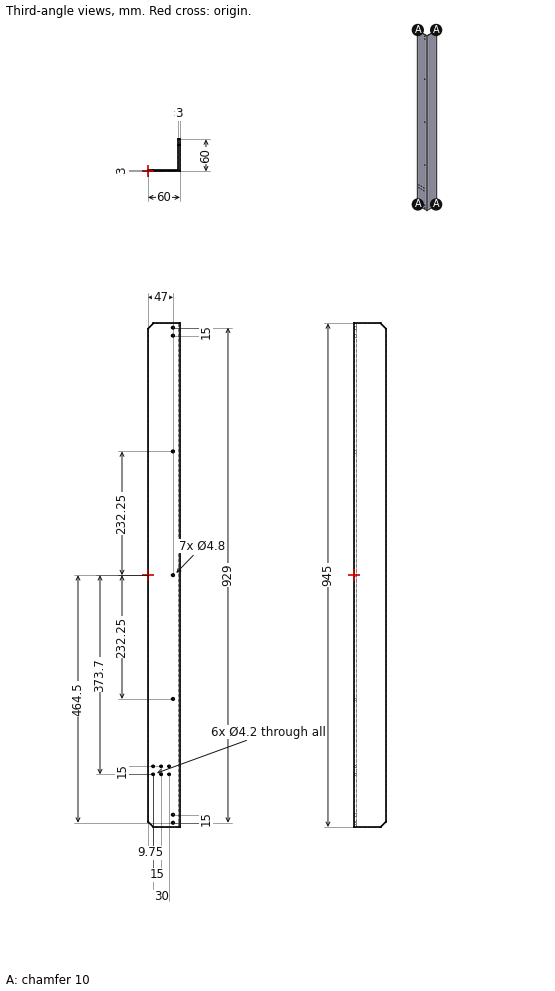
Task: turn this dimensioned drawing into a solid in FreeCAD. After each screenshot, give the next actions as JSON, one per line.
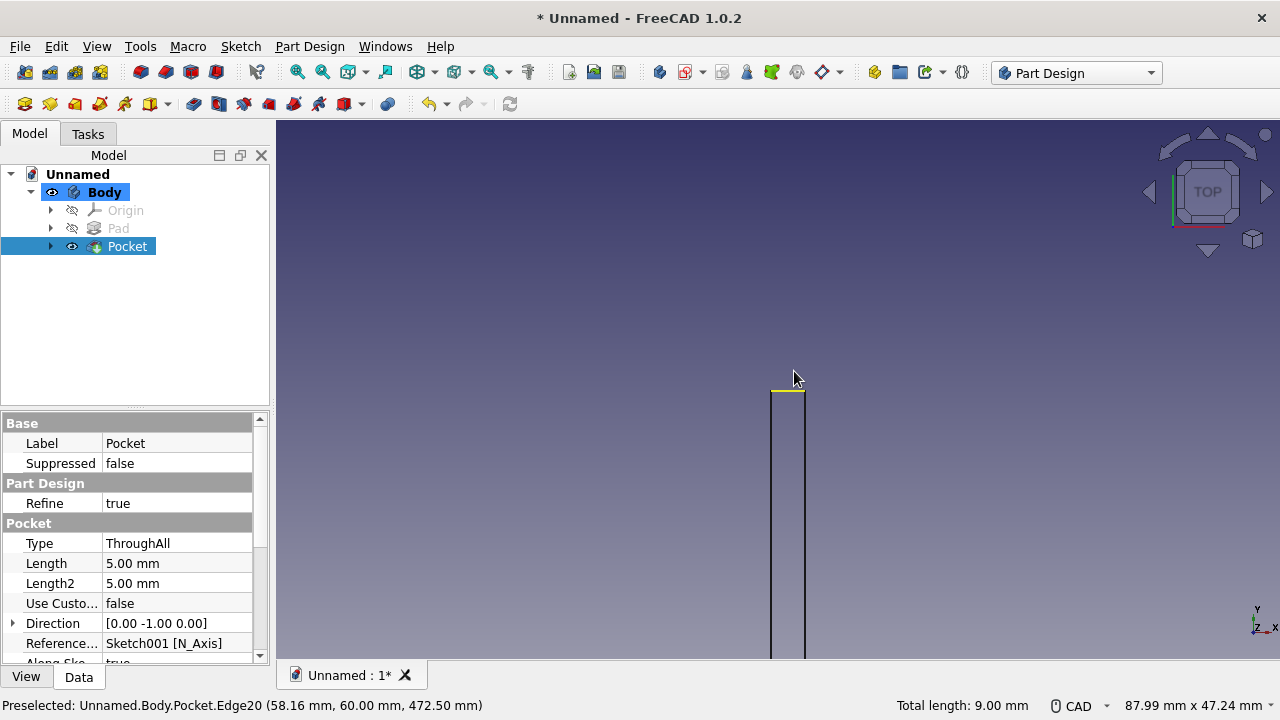
{"action": "left_click", "coordinate": [298, 72]}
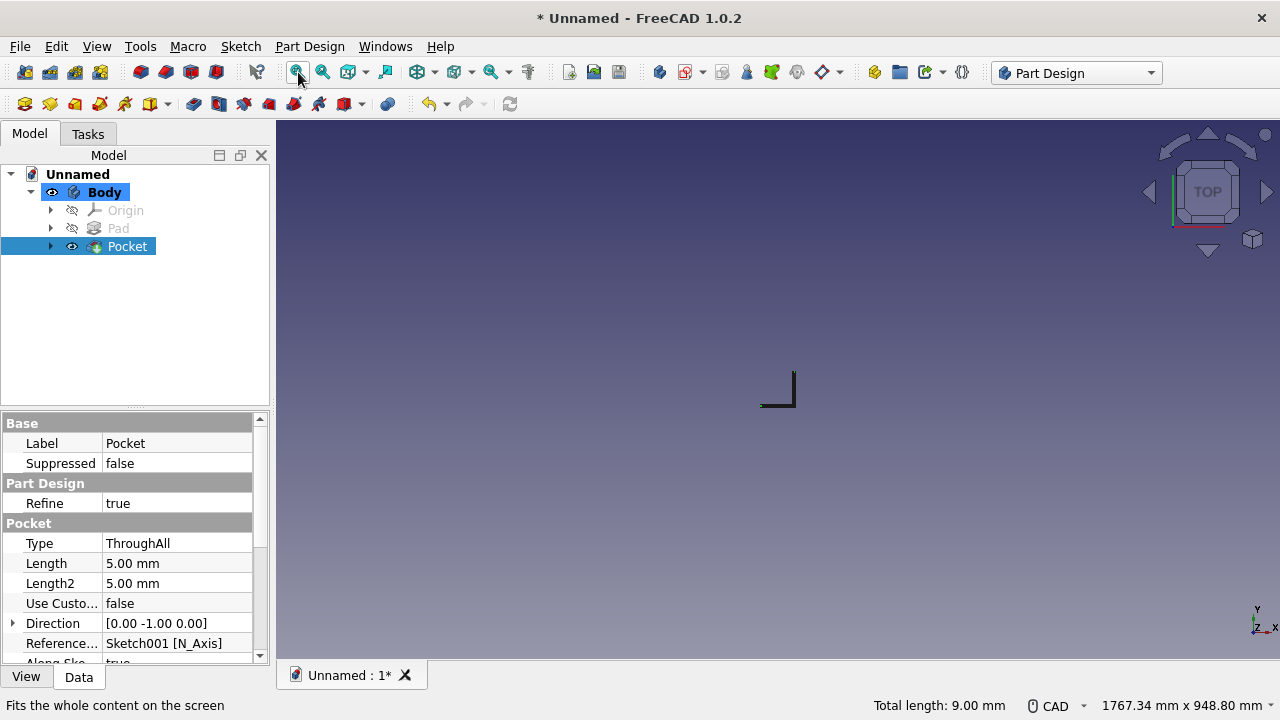
{"action": "key", "text": "1"}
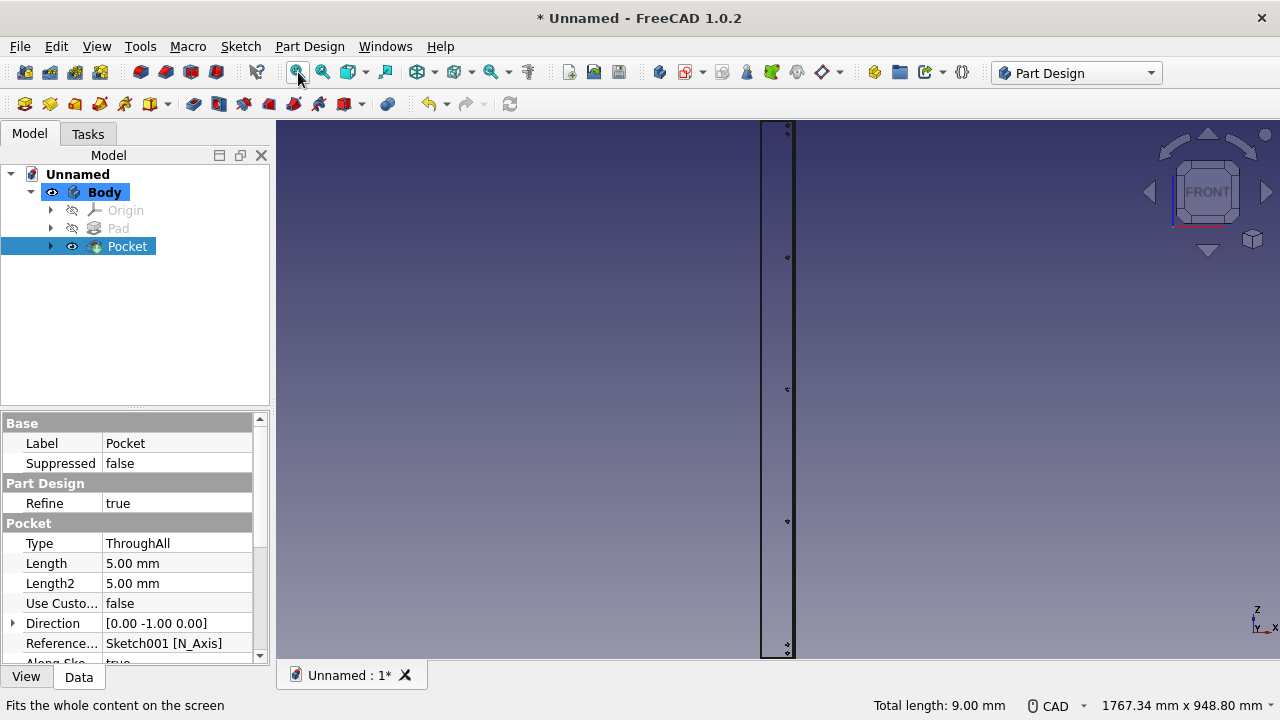
{"action": "key", "text": "3"}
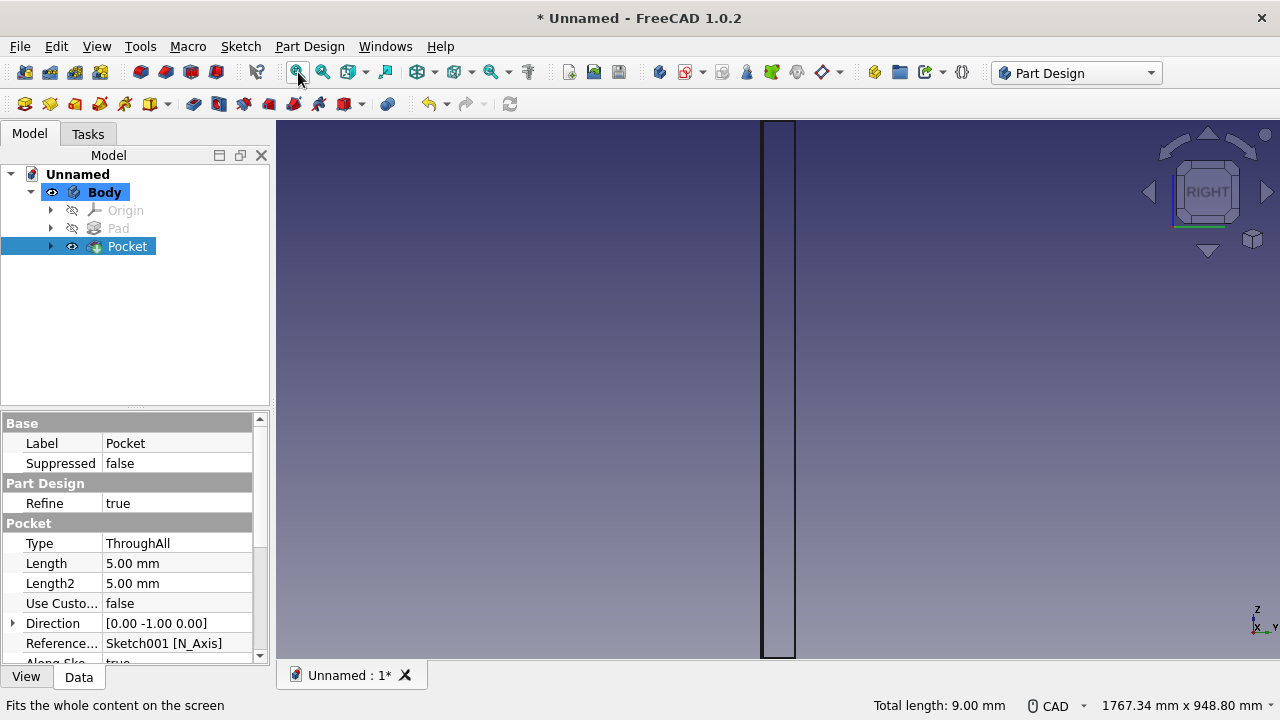
{"action": "key", "text": "5"}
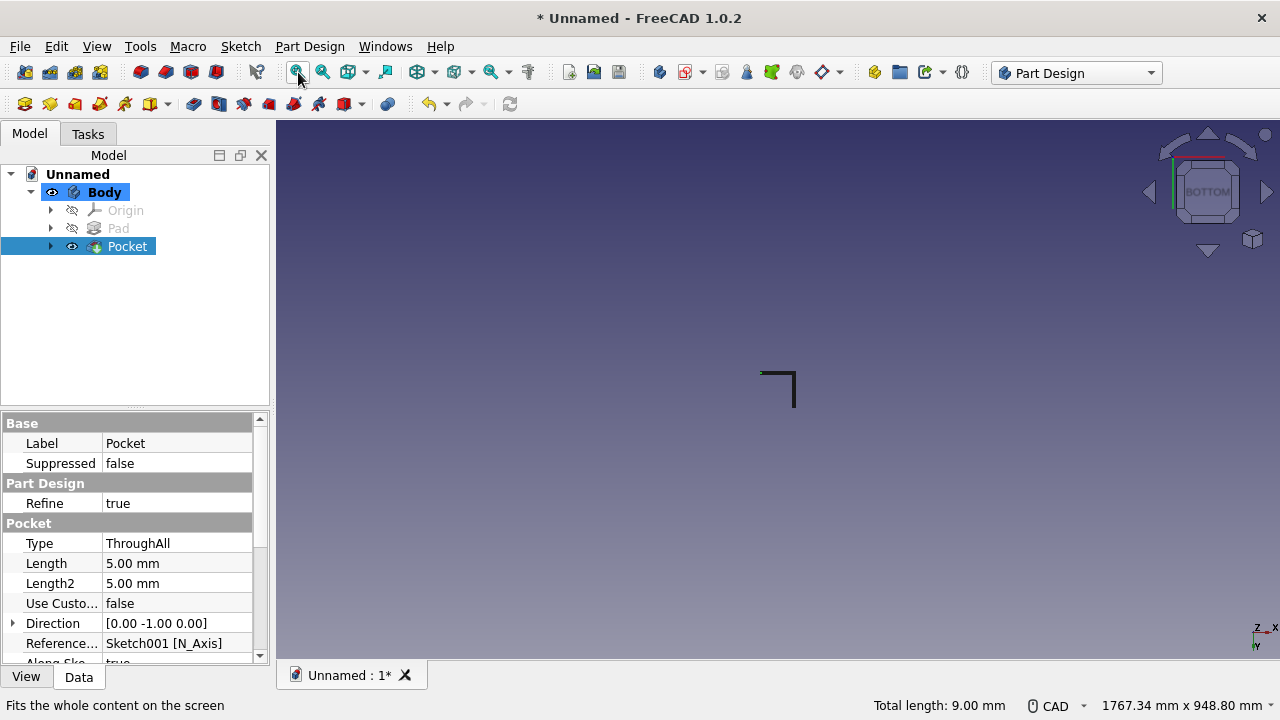
{"action": "left_click", "coordinate": [298, 72]}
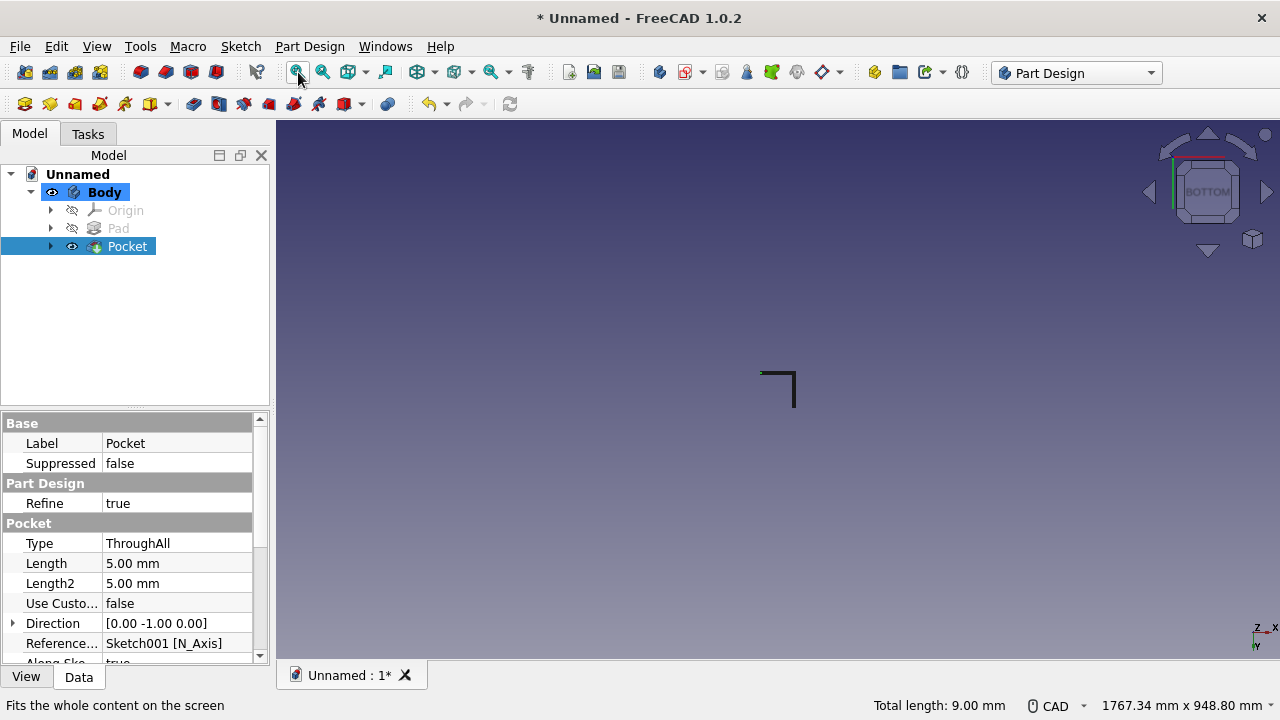
{"action": "scroll", "coordinate": [794, 406], "scroll_direction": "up", "scroll_amount": 15}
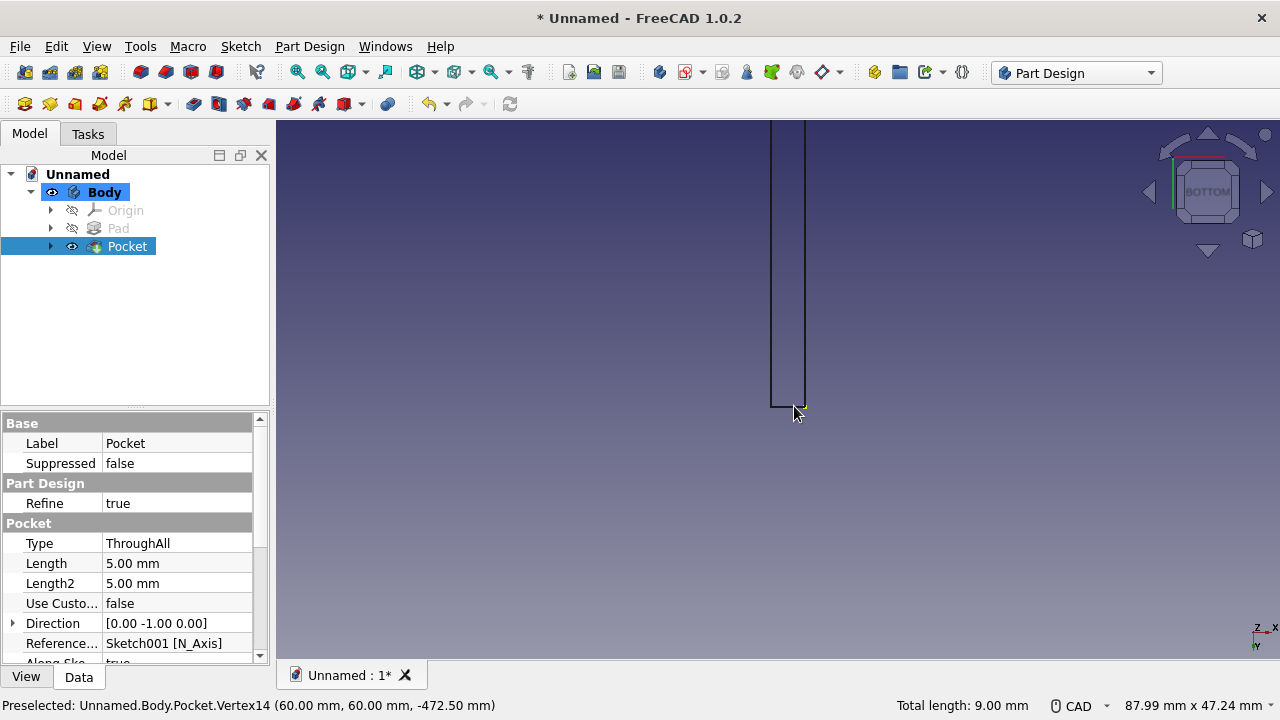
{"action": "left_click", "coordinate": [788, 406], "text": "ctrl"}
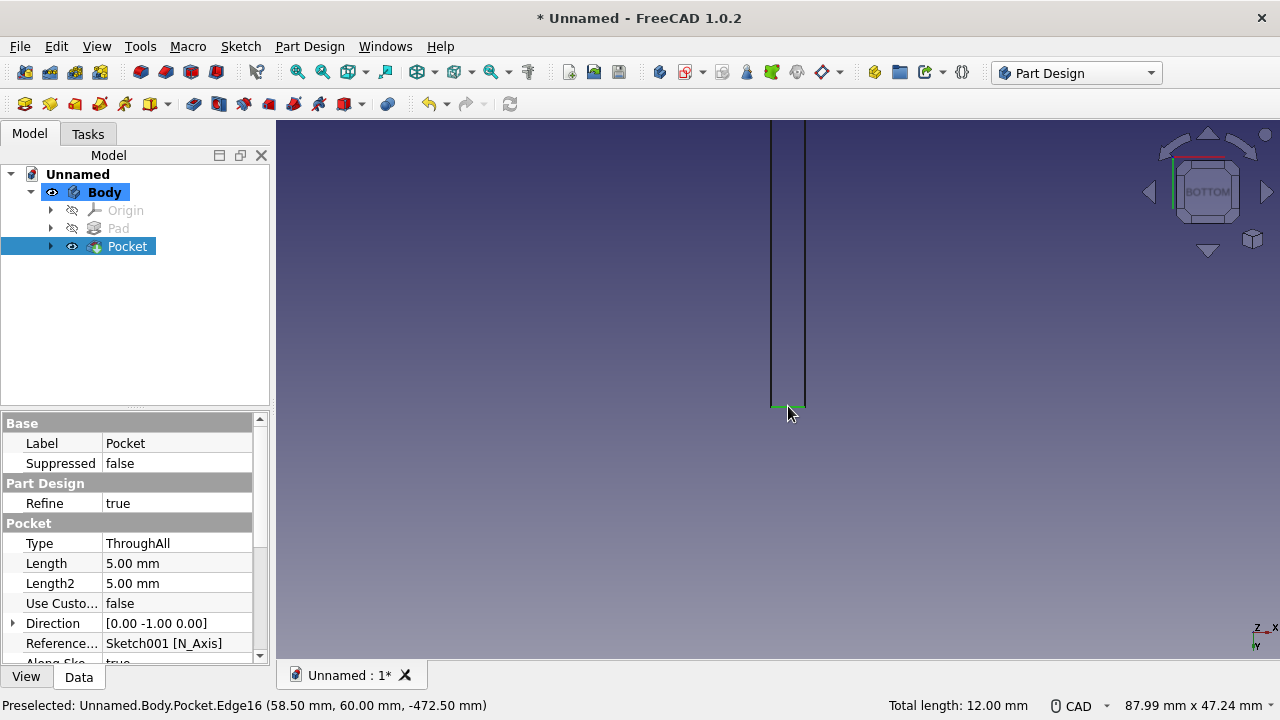
{"action": "key", "text": "v 1"}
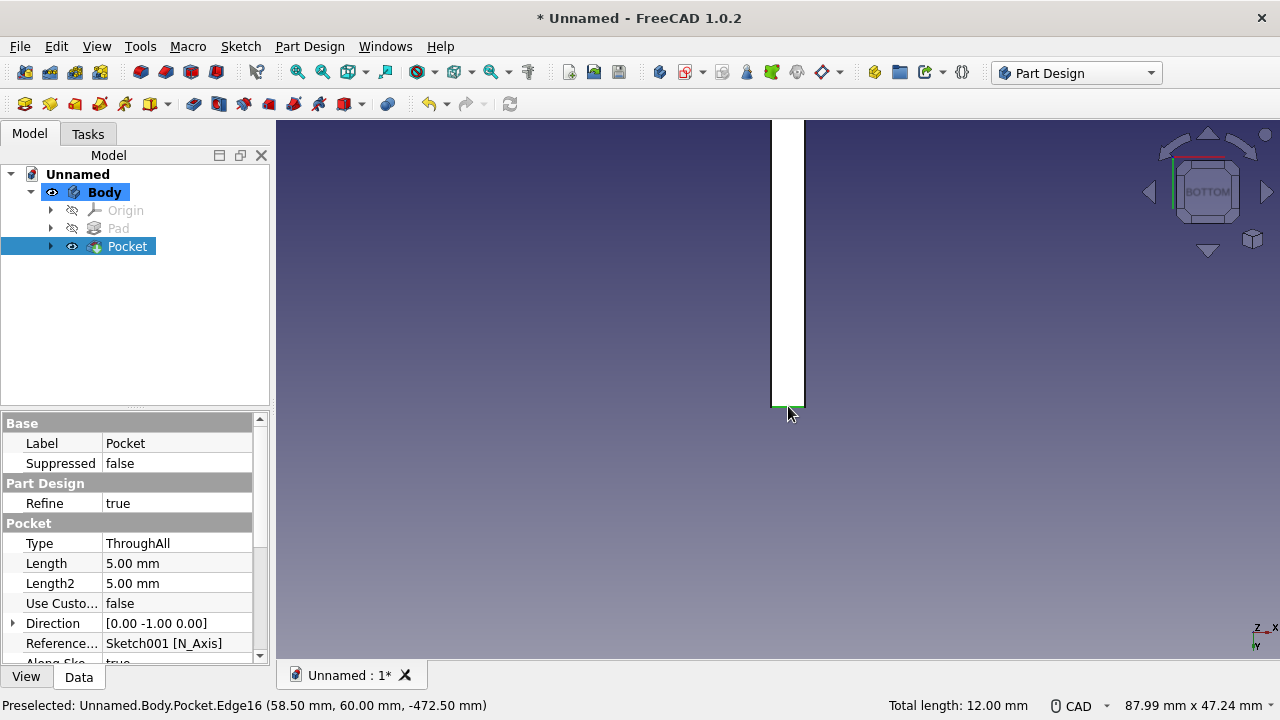
{"action": "left_click", "coordinate": [166, 72]}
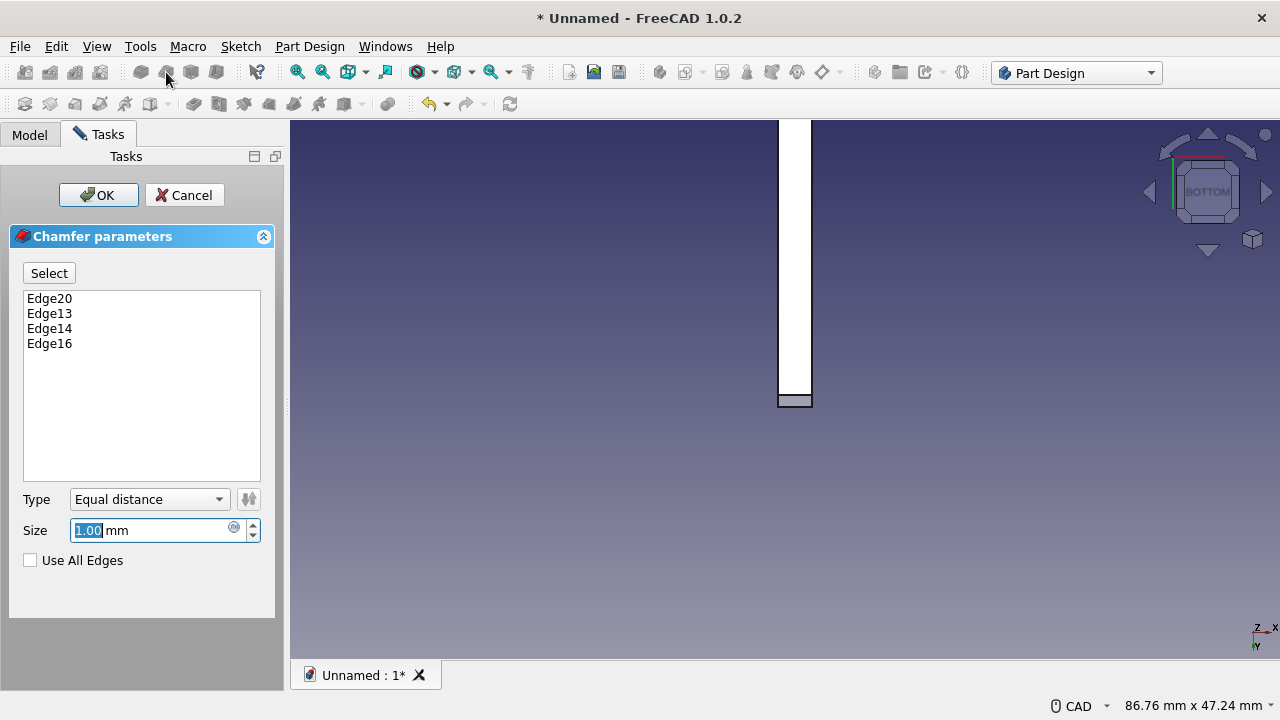
{"action": "type", "text": "10"}
{"action": "key", "text": "Tab"}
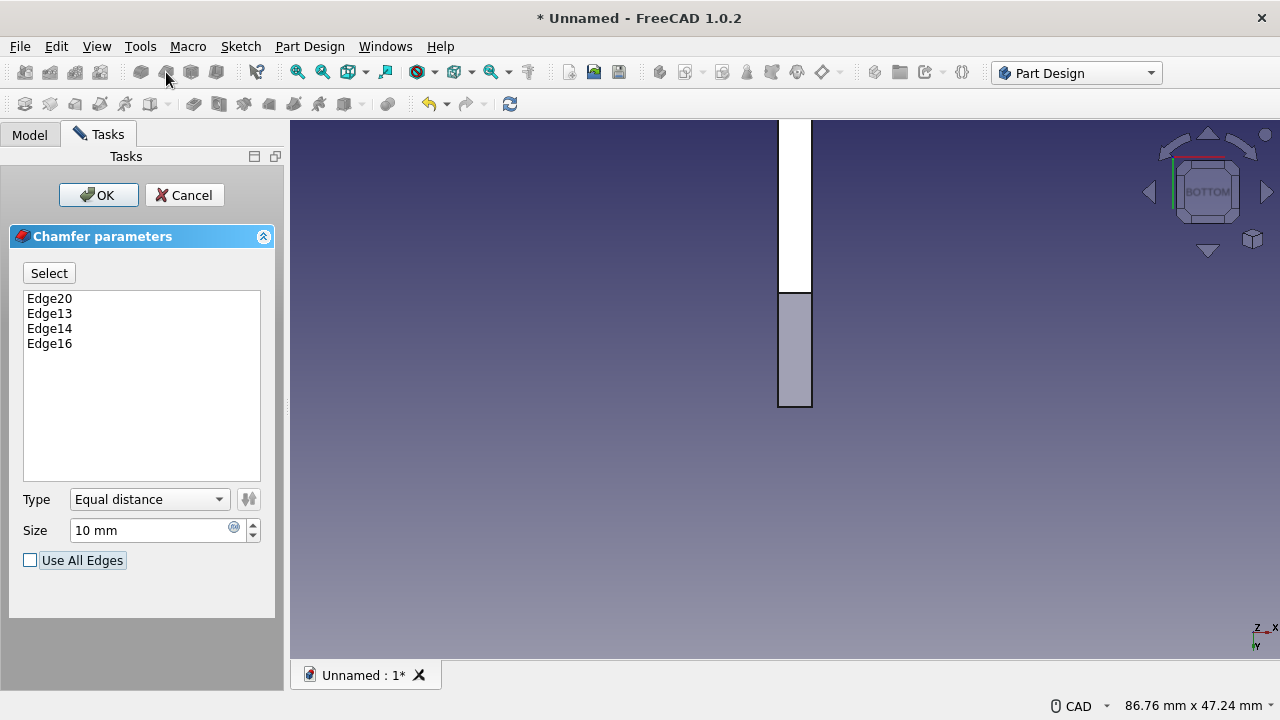
{"action": "left_click", "coordinate": [99, 195]}